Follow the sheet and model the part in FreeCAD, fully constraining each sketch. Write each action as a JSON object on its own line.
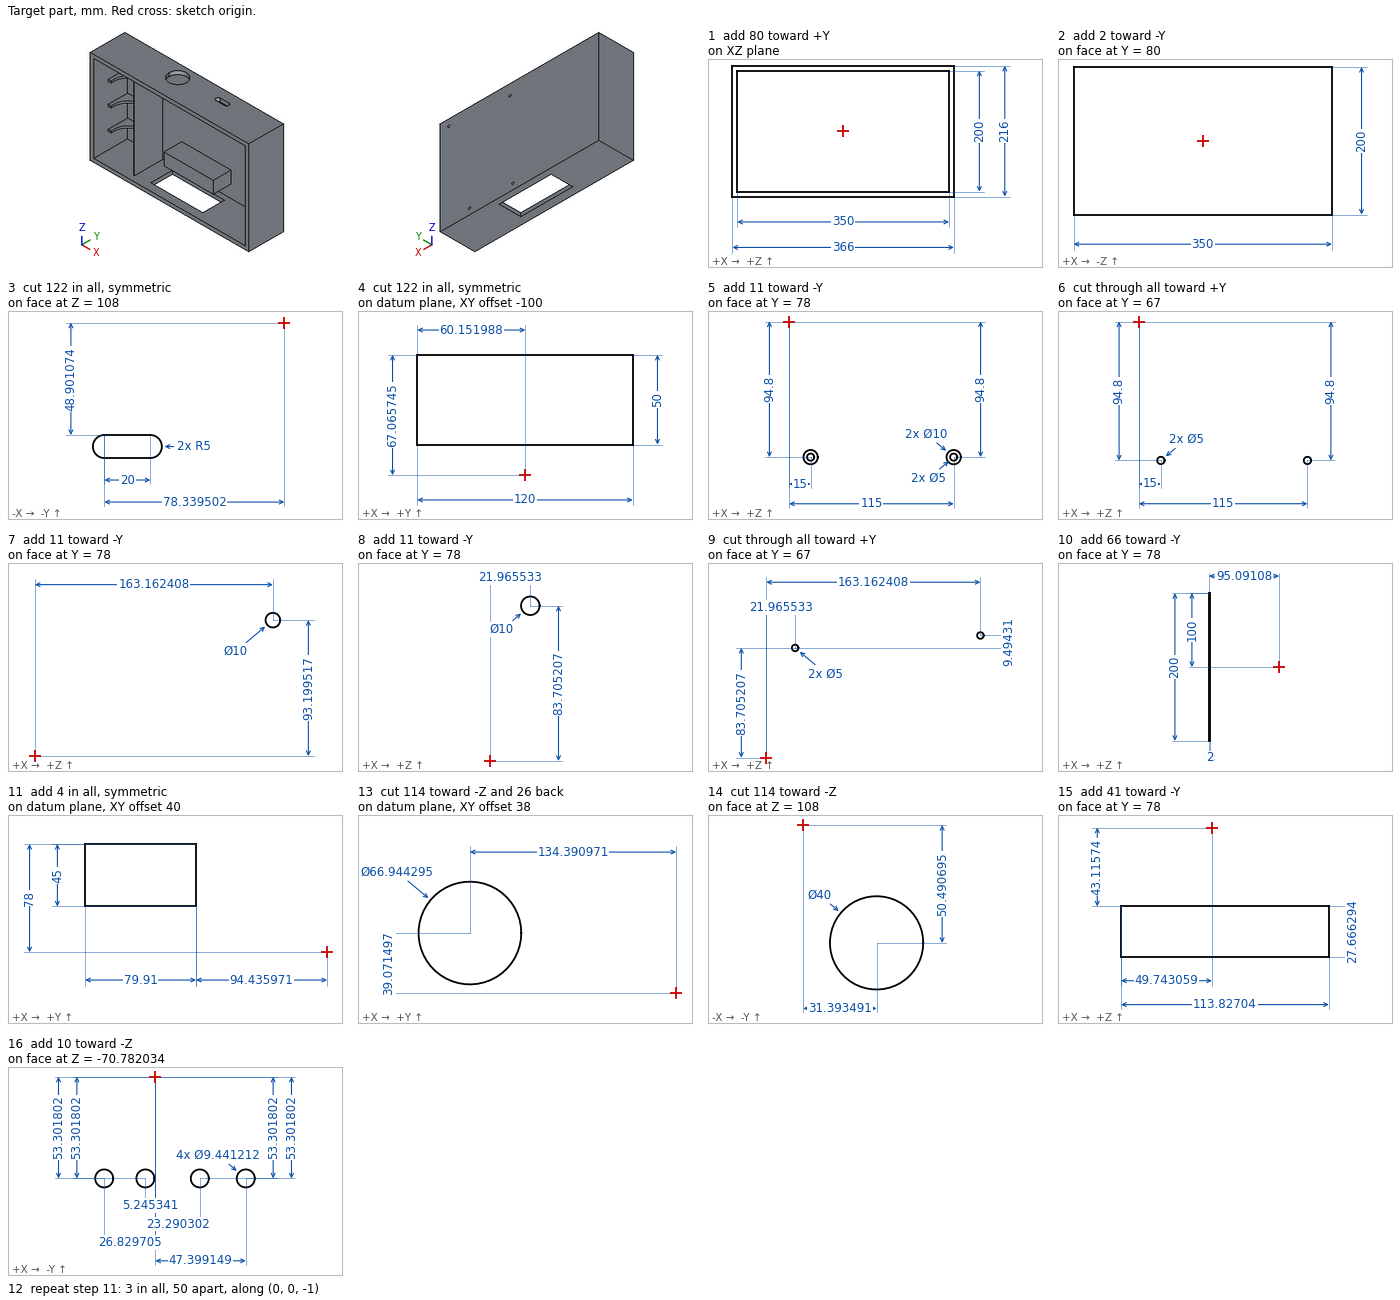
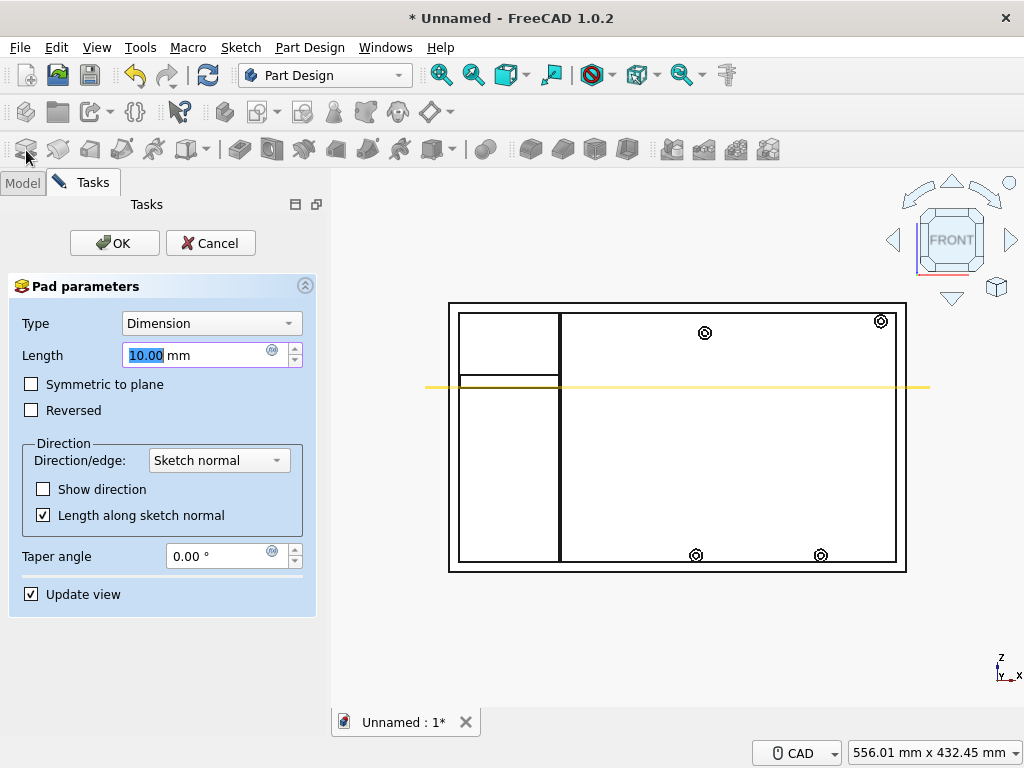
{"action": "type", "text": "4"}
{"action": "key", "text": "Tab"}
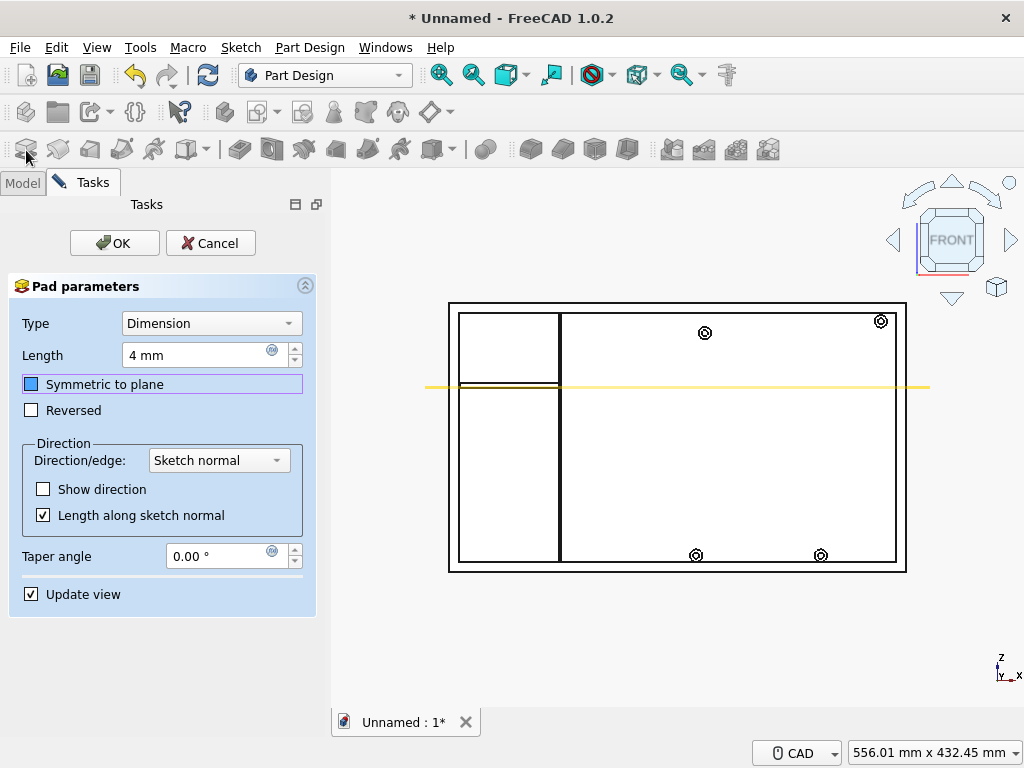
{"action": "left_click", "coordinate": [30, 384]}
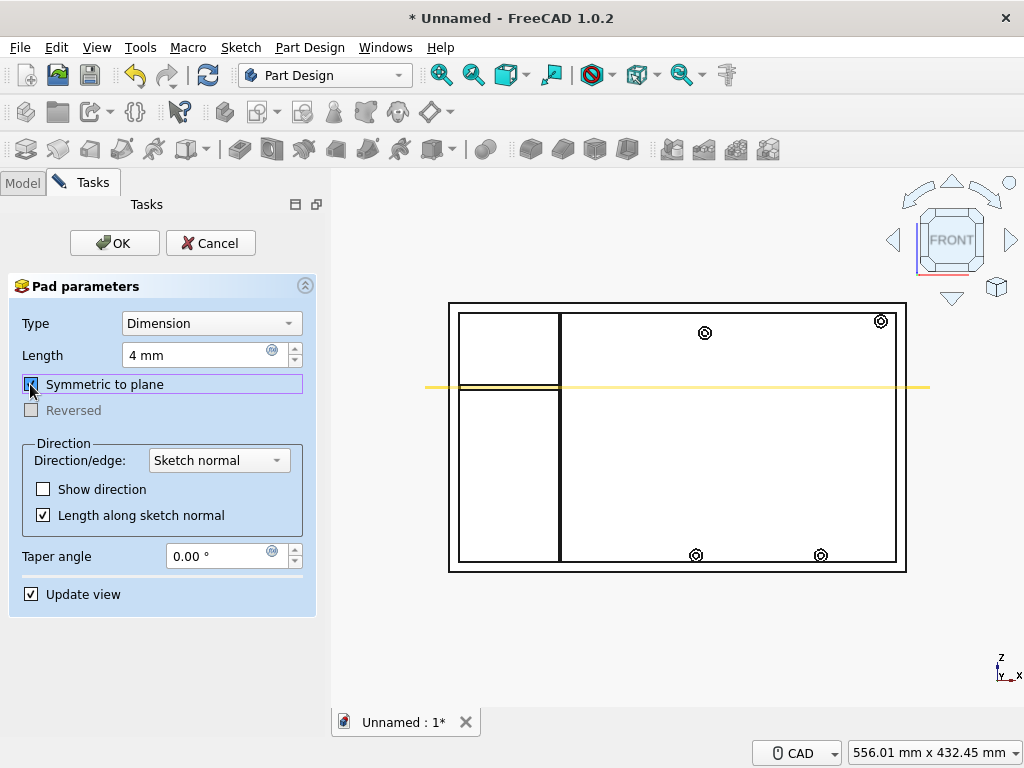
{"action": "left_click", "coordinate": [115, 243]}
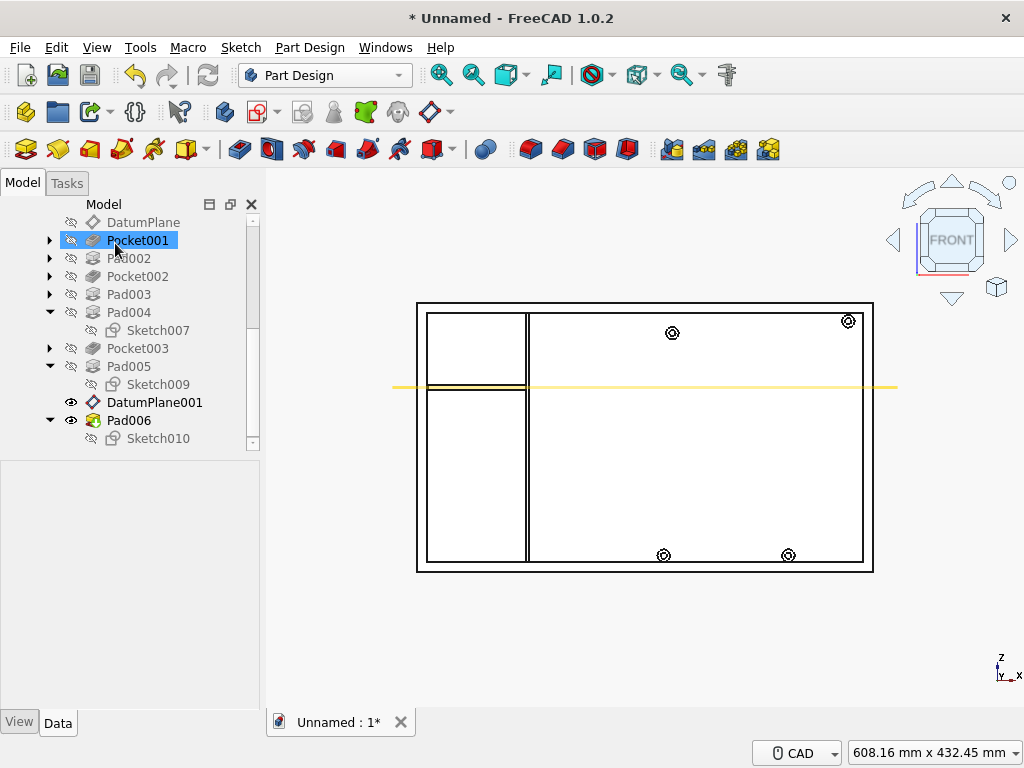
{"action": "left_click", "coordinate": [116, 402]}
{"action": "key", "text": "space"}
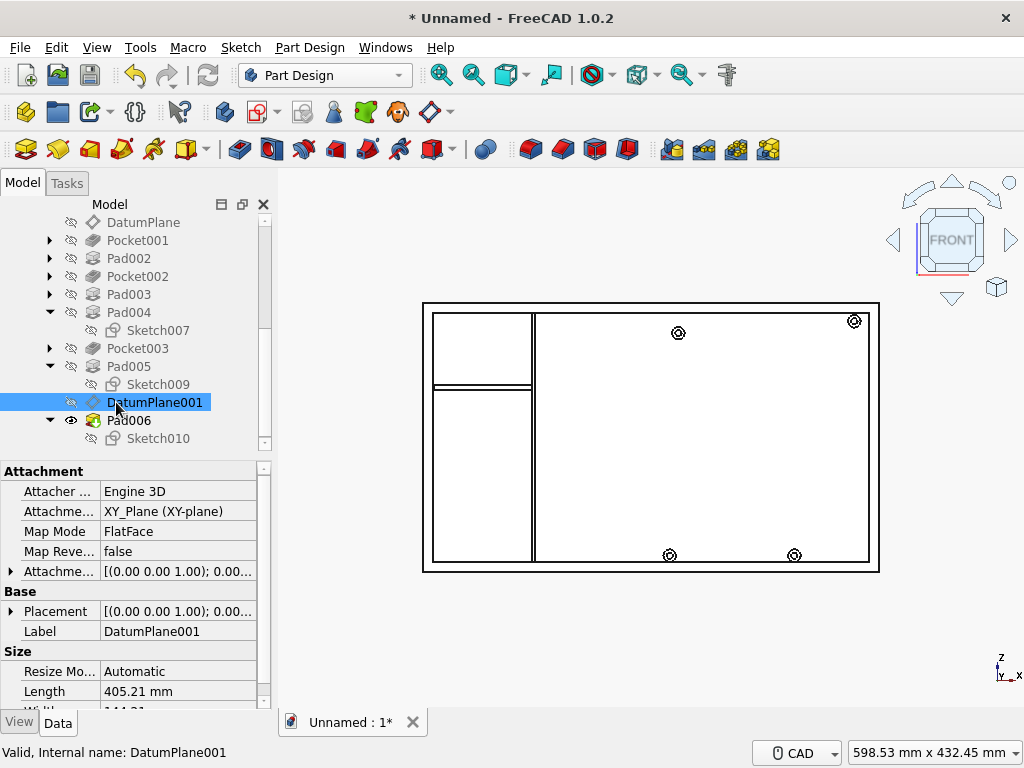
{"action": "left_click", "coordinate": [116, 420]}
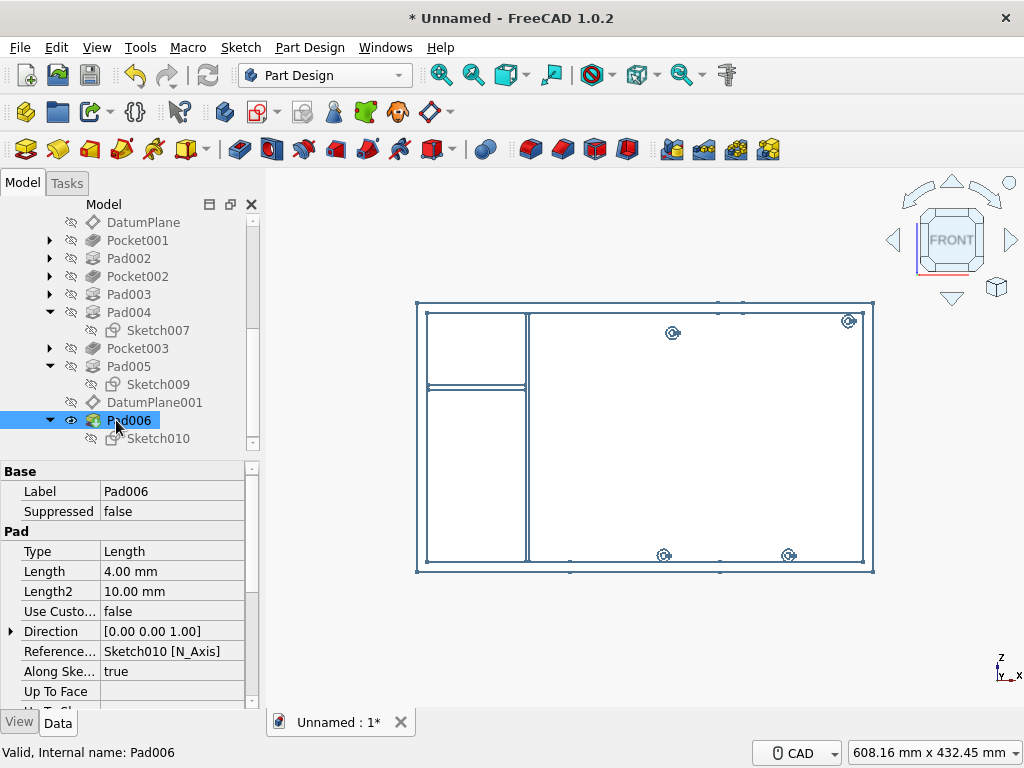
{"action": "left_click", "coordinate": [704, 150]}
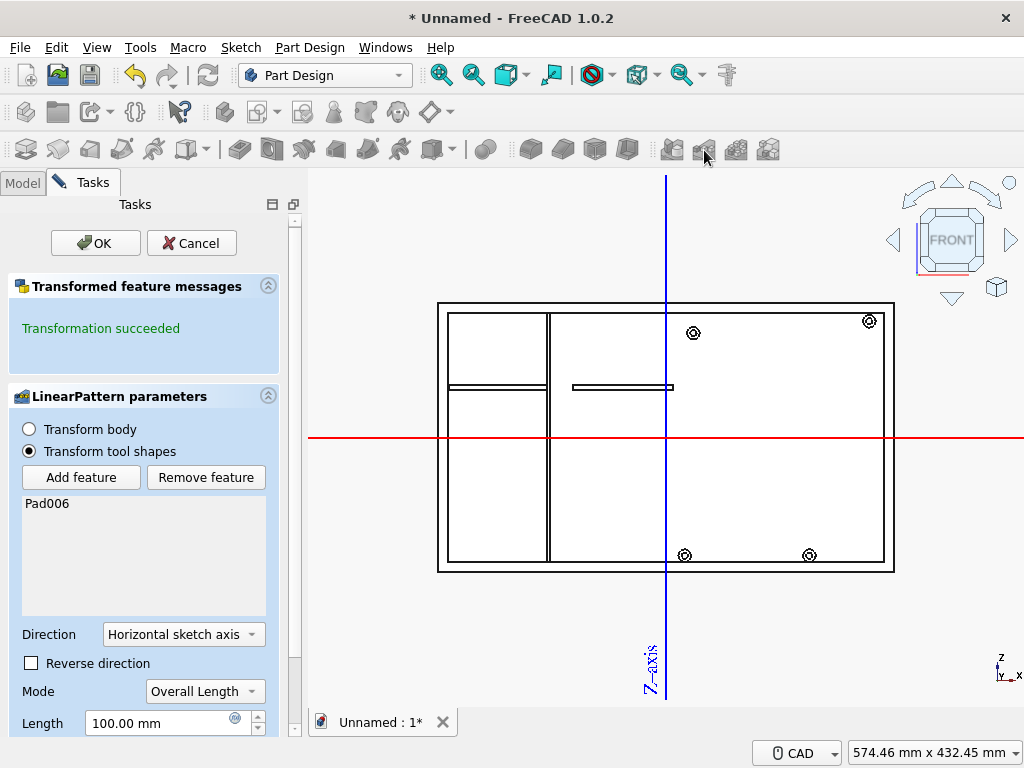
{"action": "left_click", "coordinate": [184, 634]}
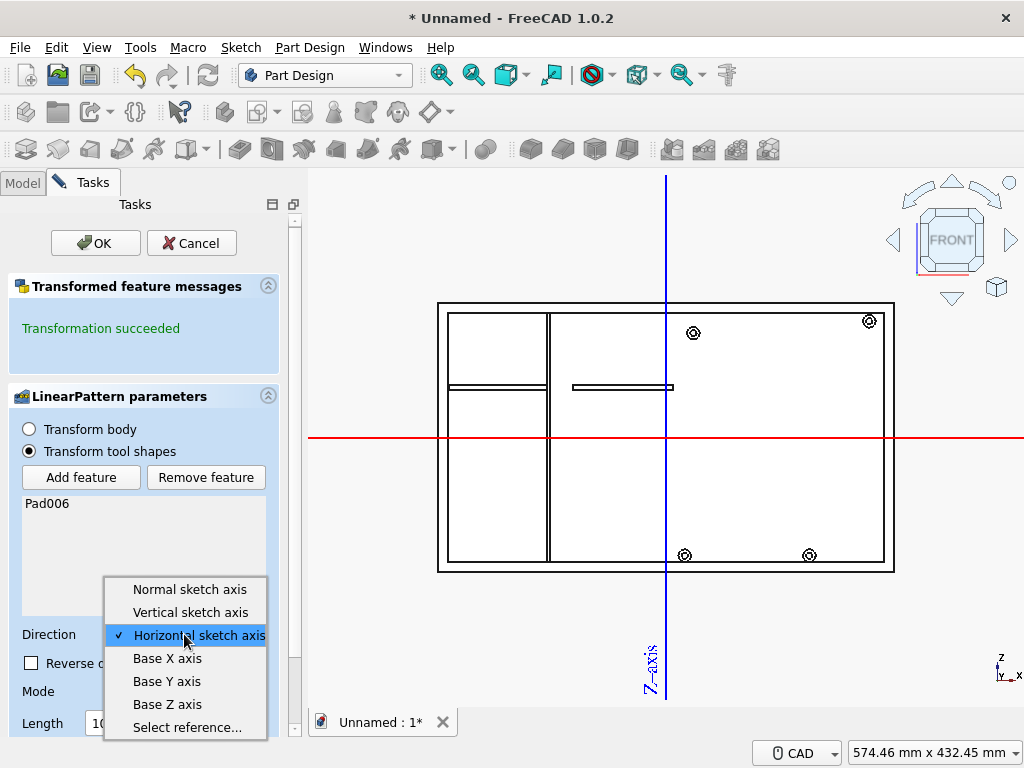
{"action": "left_click", "coordinate": [184, 704]}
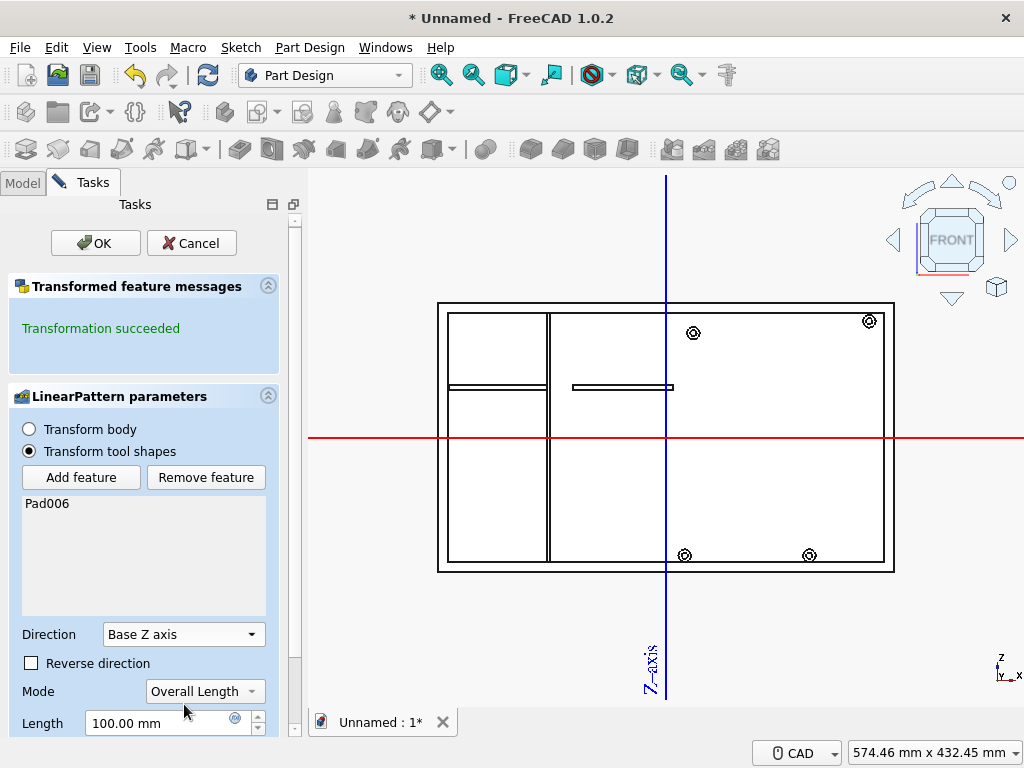
{"action": "left_click", "coordinate": [206, 692]}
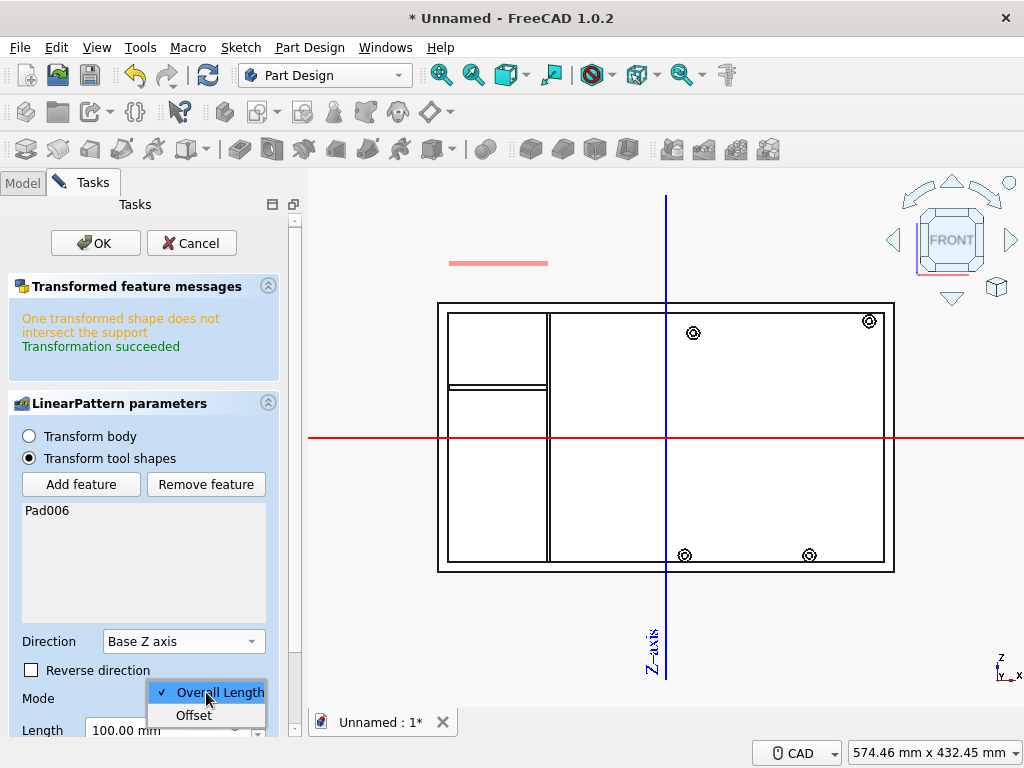
{"action": "left_click", "coordinate": [206, 716]}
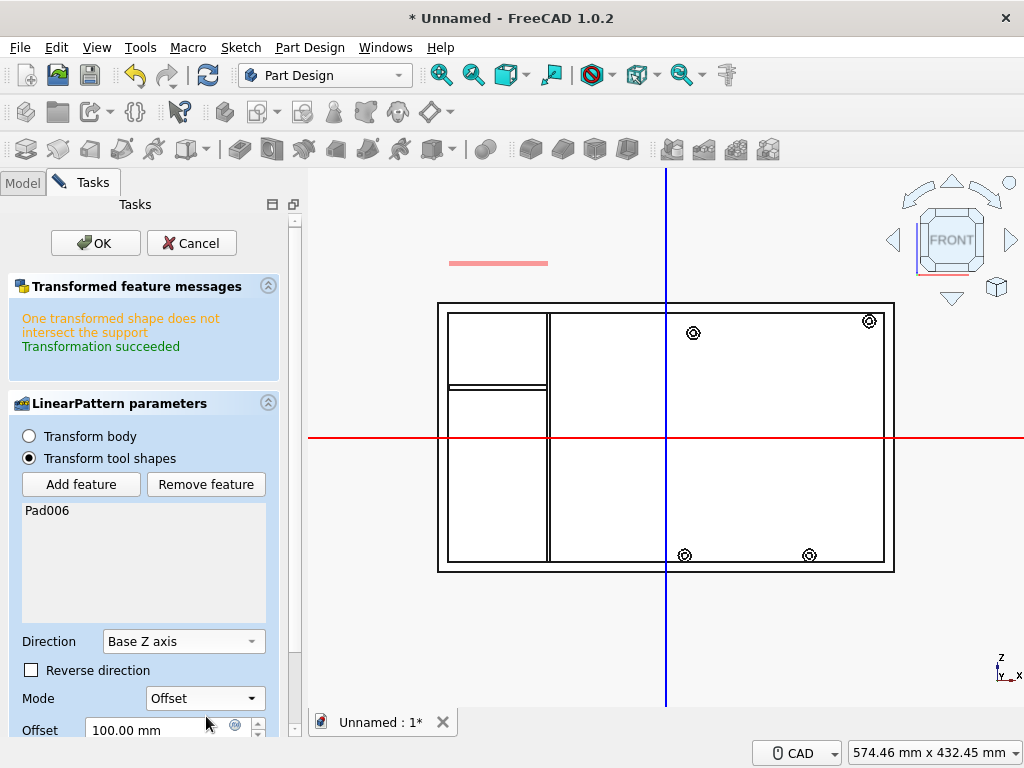
{"action": "scroll", "coordinate": [295, 475], "scroll_direction": "down", "scroll_amount": 2}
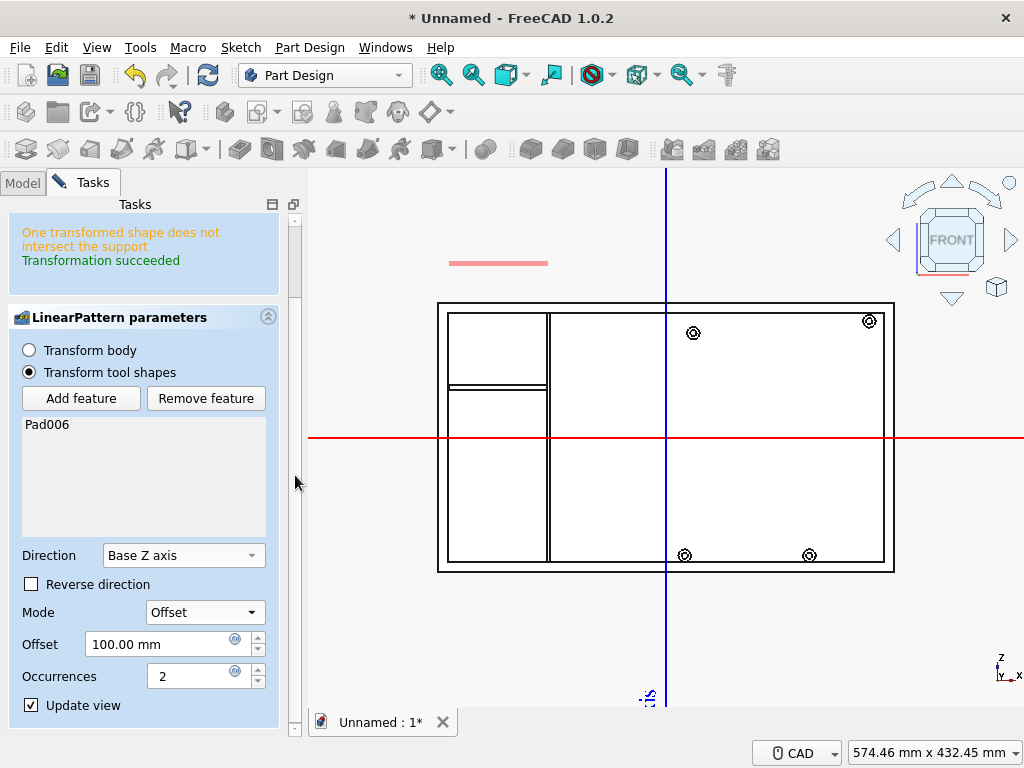
{"action": "triple_click", "coordinate": [168, 644]}